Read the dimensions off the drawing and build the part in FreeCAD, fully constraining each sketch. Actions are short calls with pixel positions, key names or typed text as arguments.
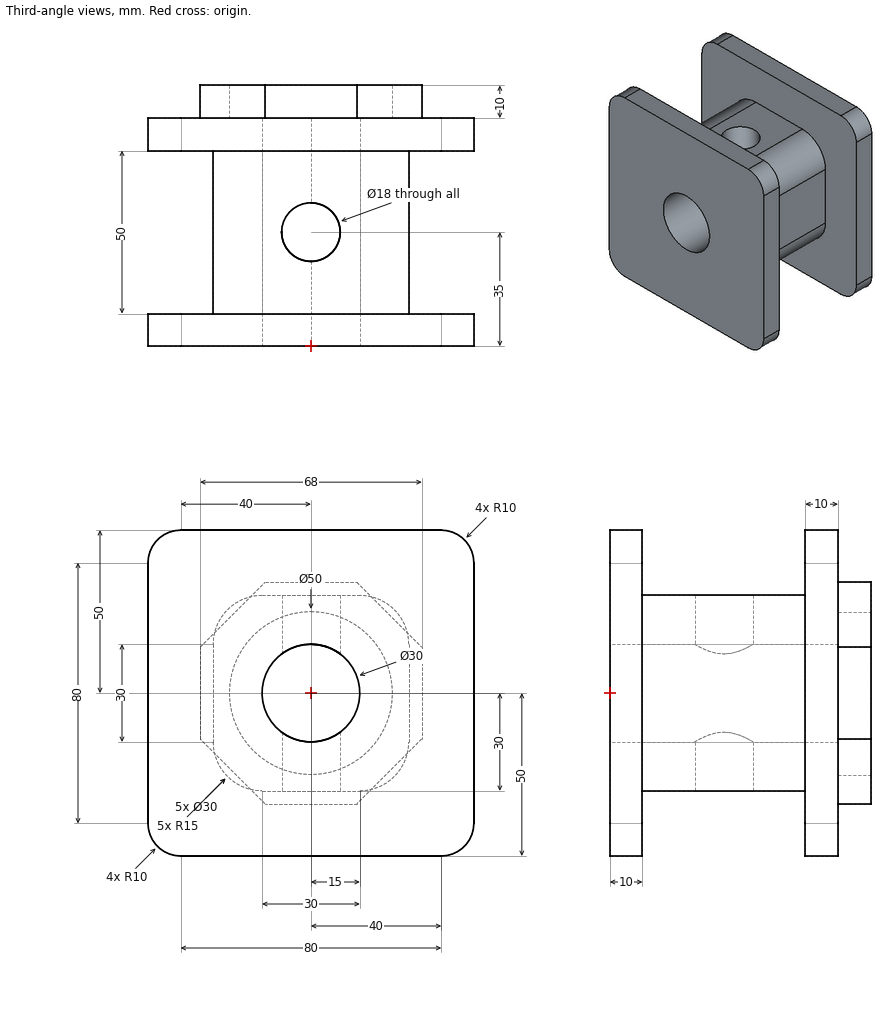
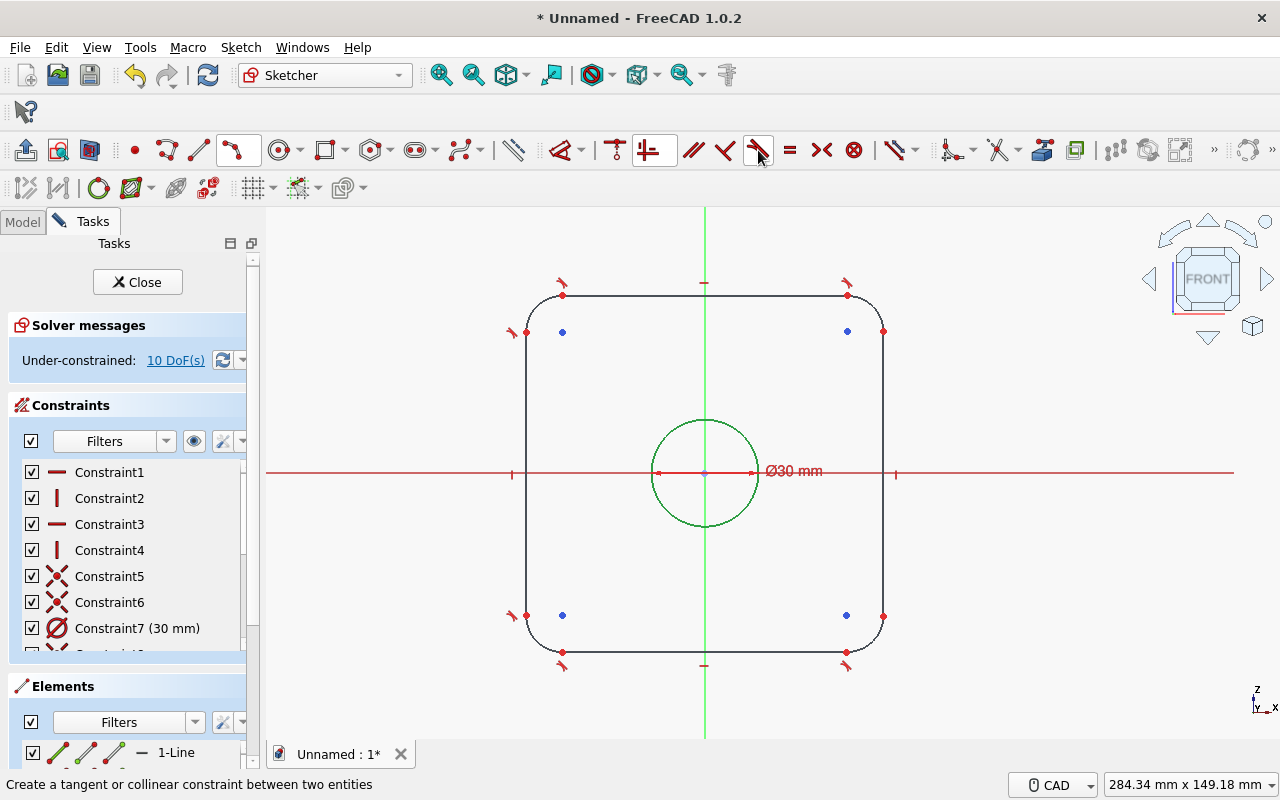
click(883, 418)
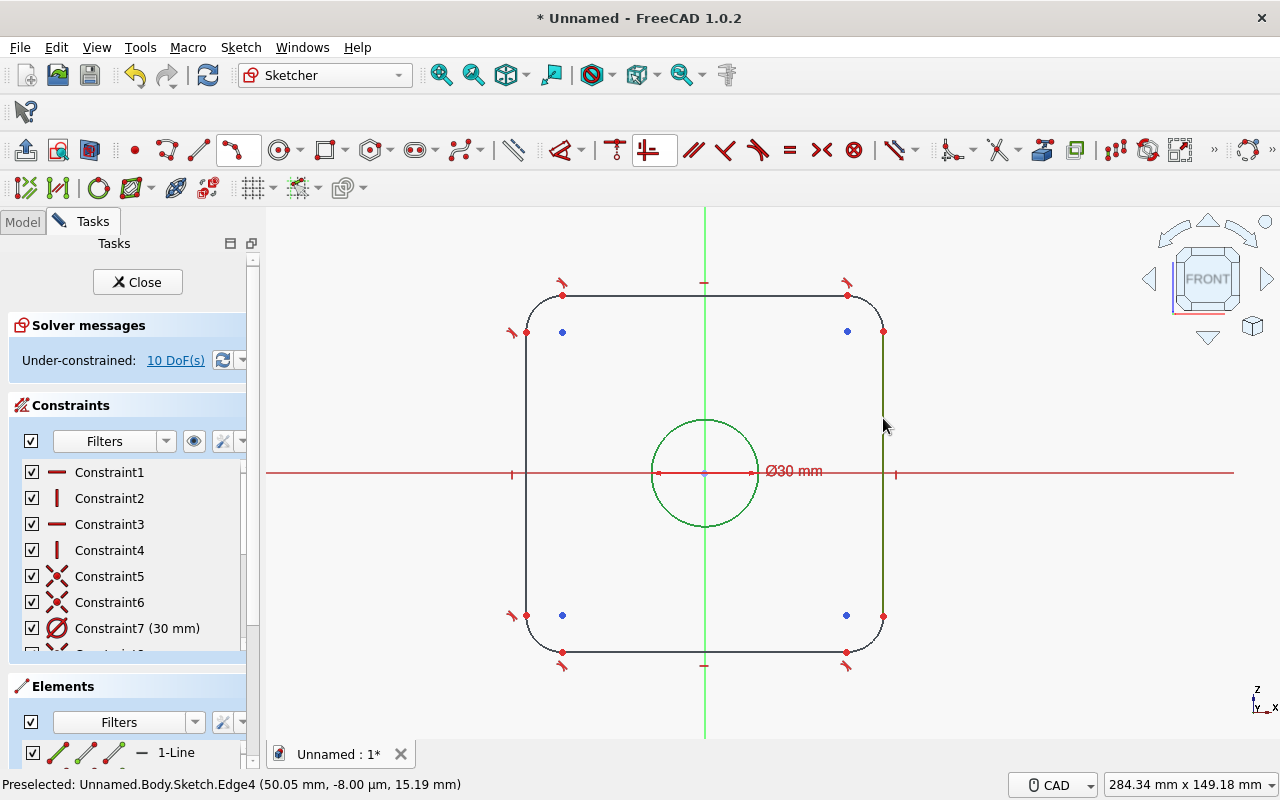
click(880, 316)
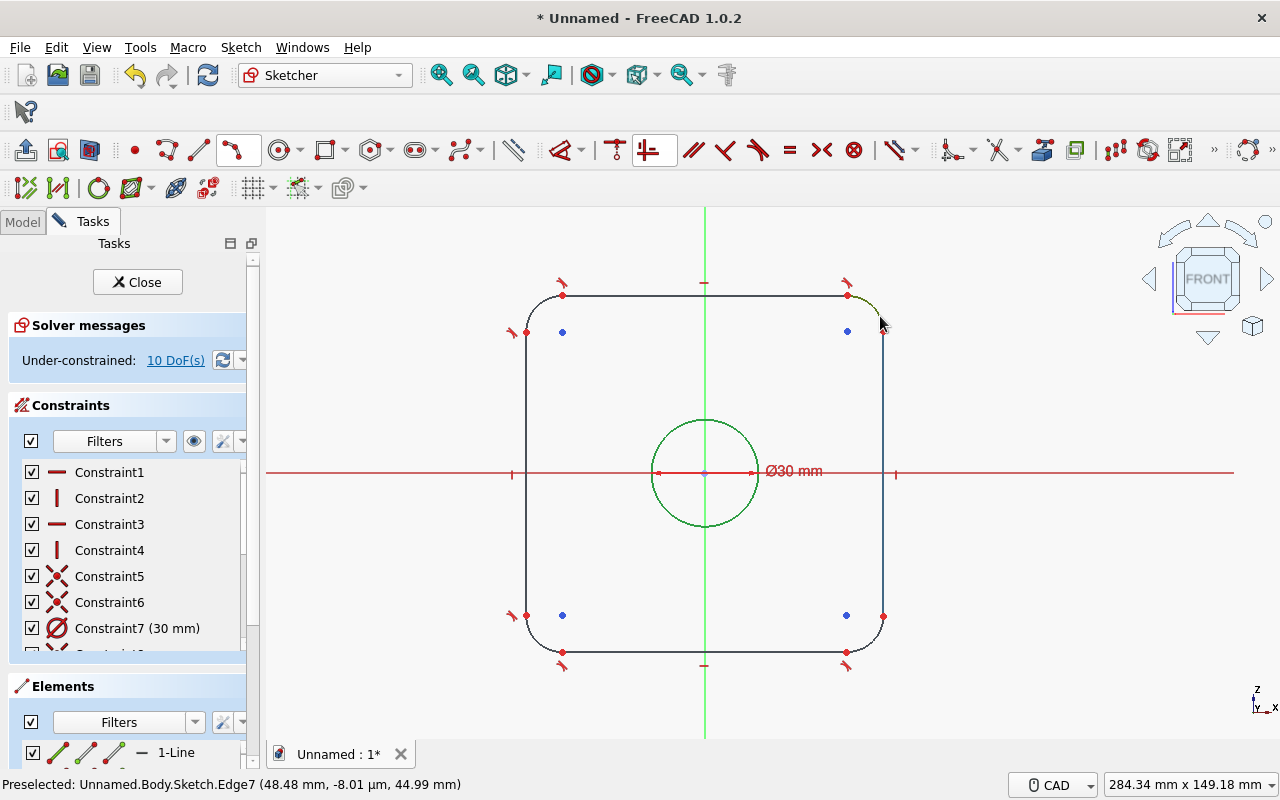
click(758, 150)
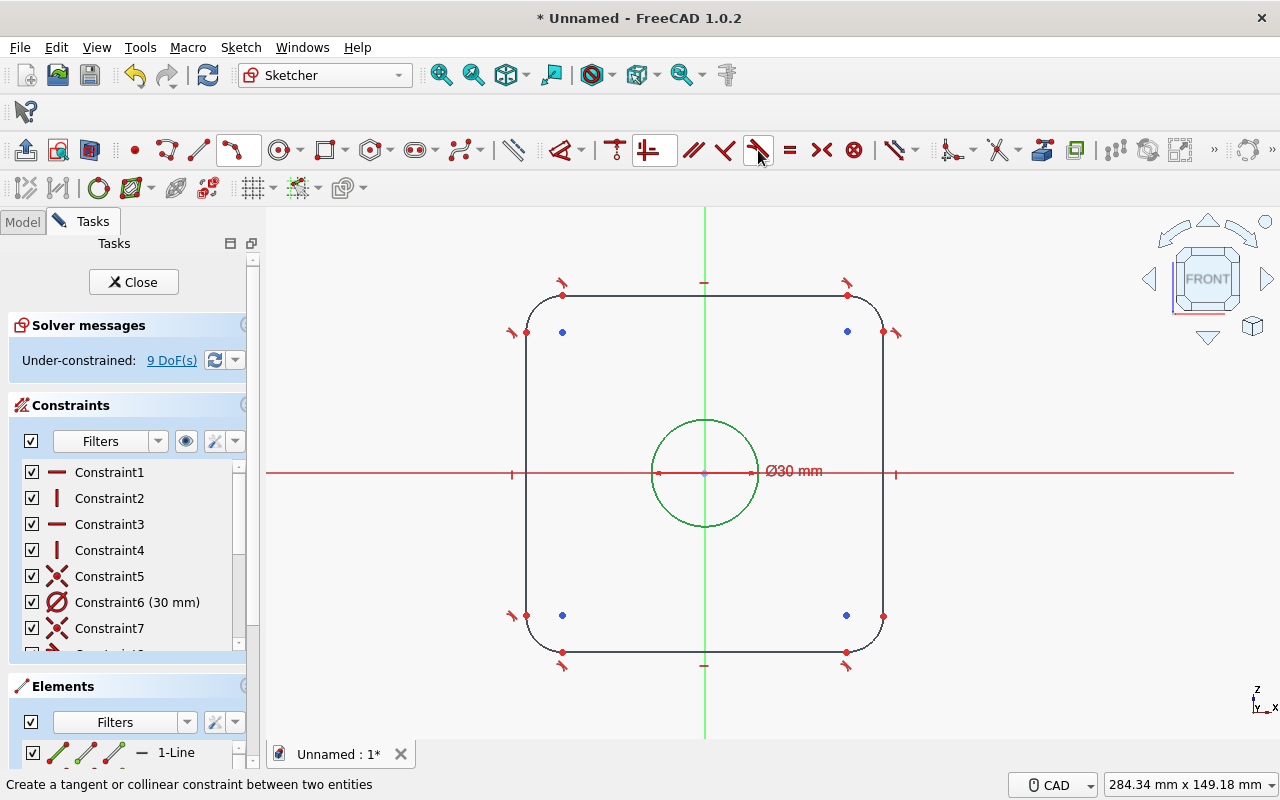
click(883, 418)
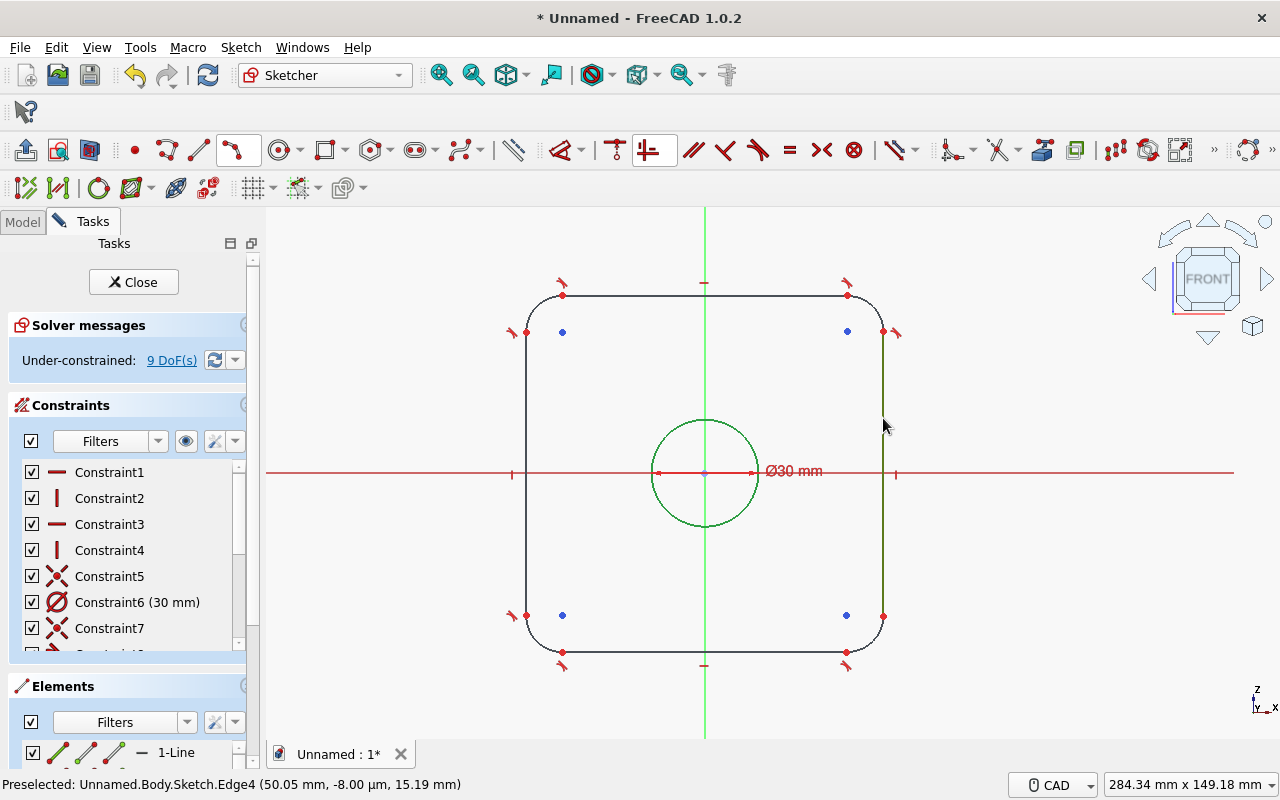
click(863, 648)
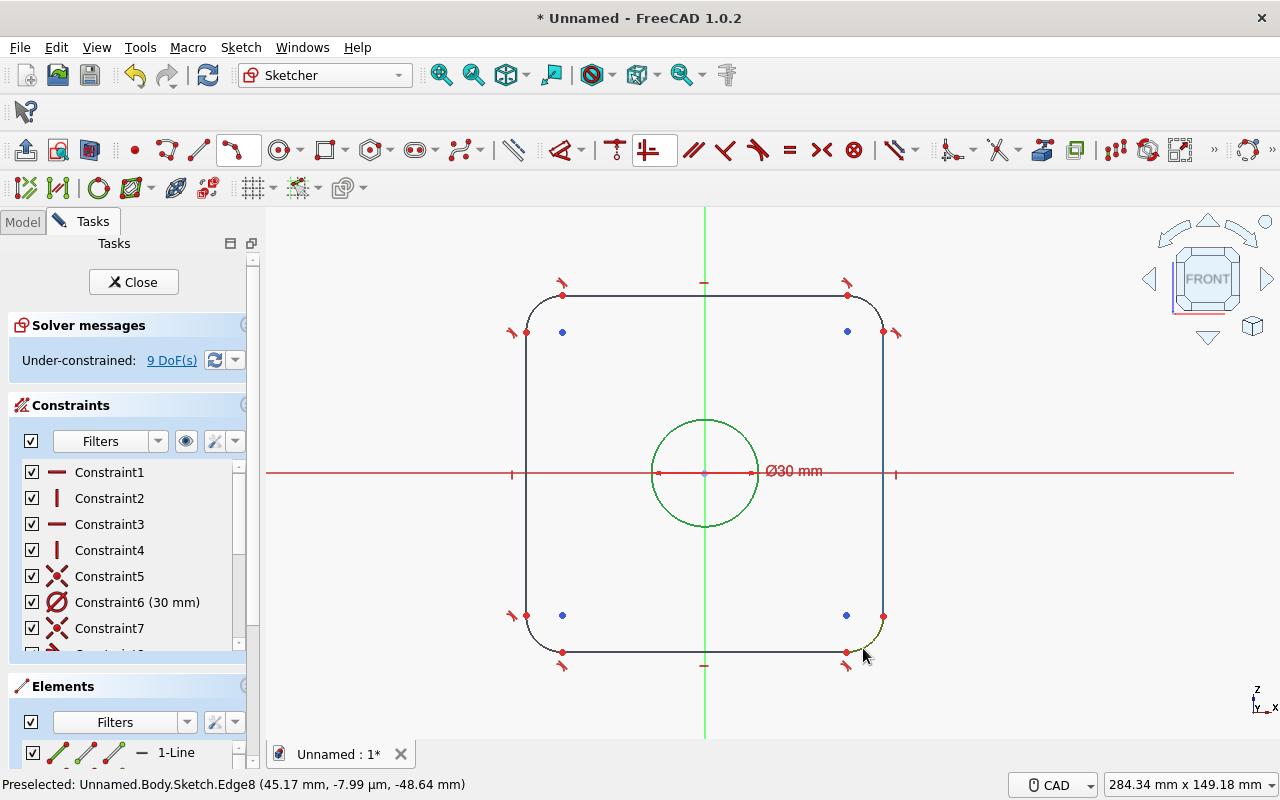
click(758, 150)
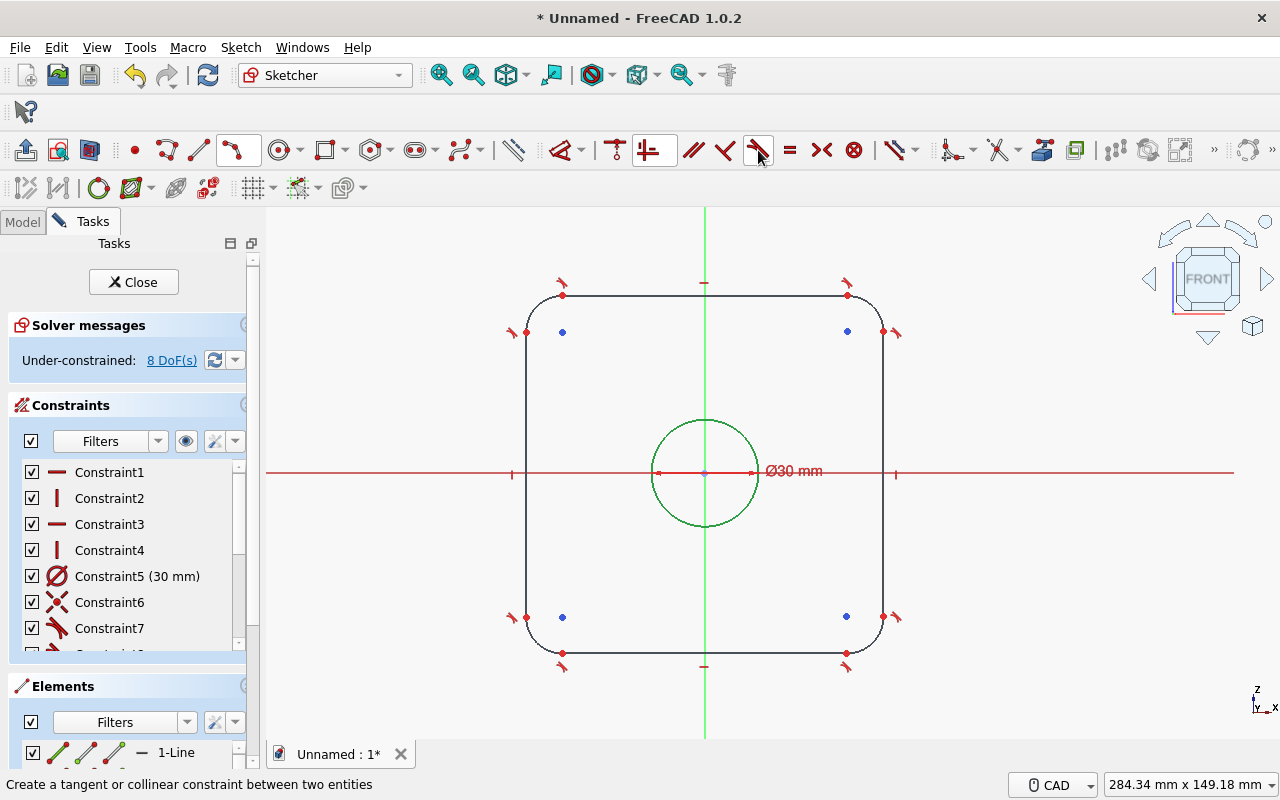
click(530, 634)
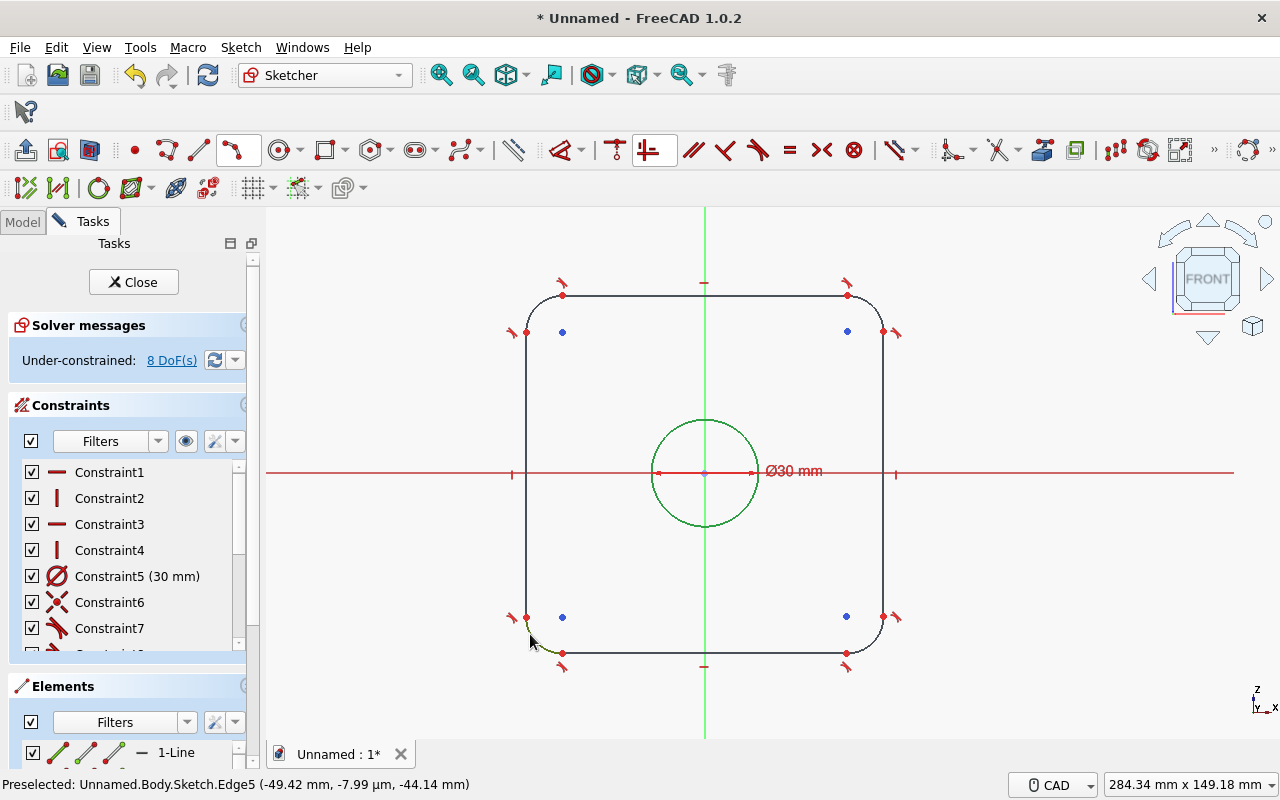
click(546, 300)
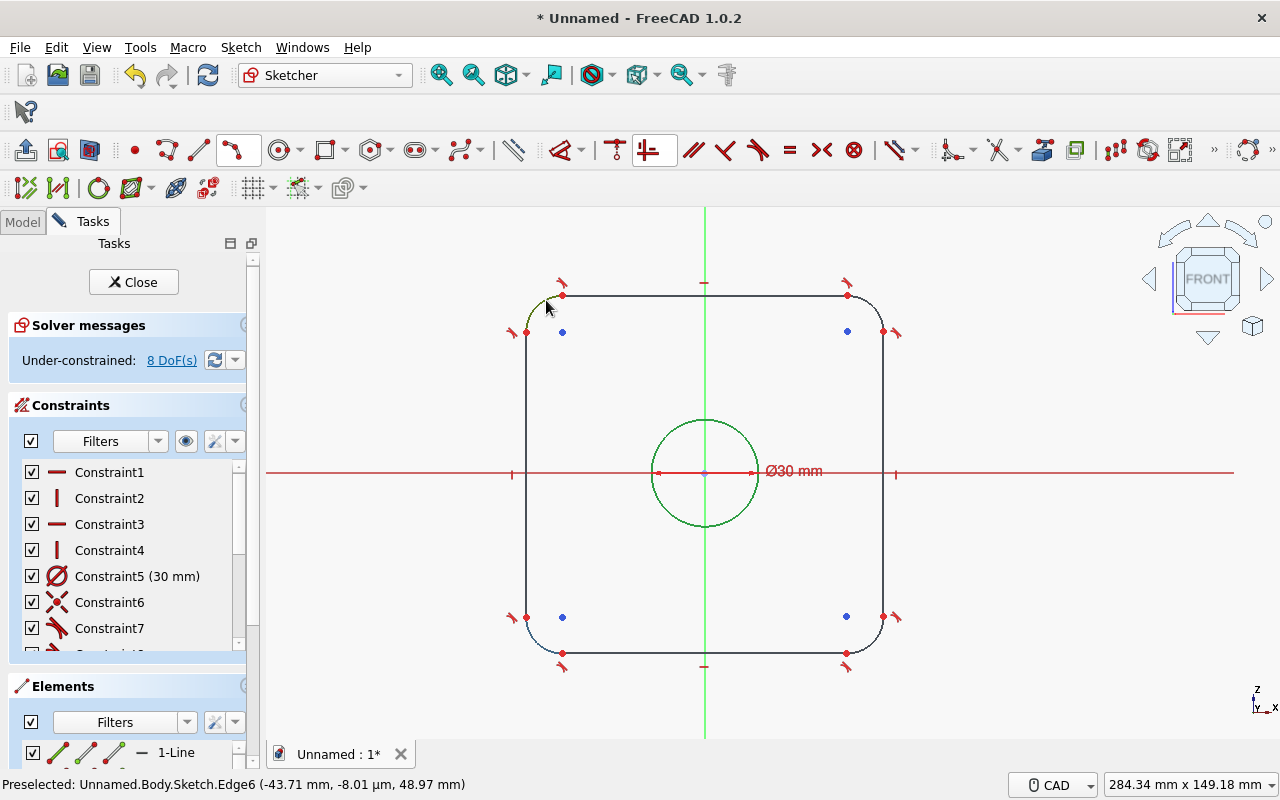
click(880, 316)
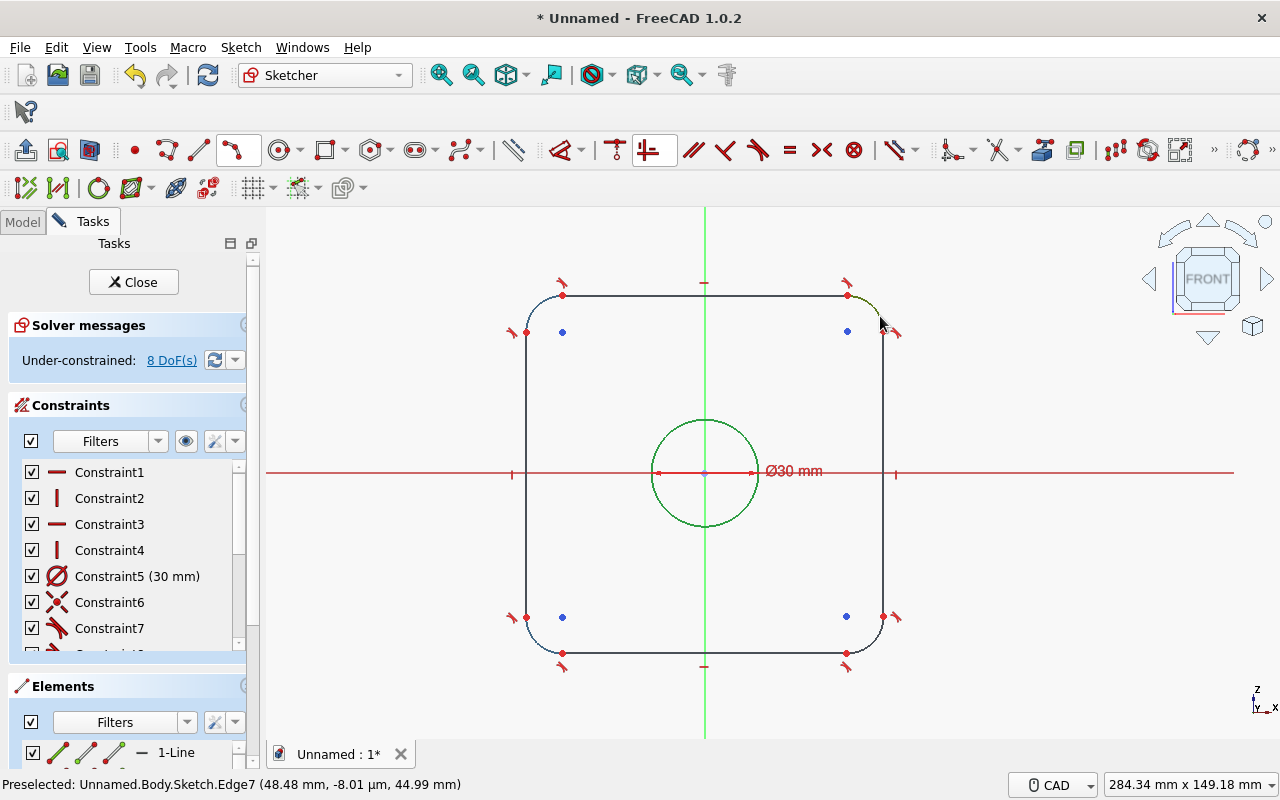
click(864, 650)